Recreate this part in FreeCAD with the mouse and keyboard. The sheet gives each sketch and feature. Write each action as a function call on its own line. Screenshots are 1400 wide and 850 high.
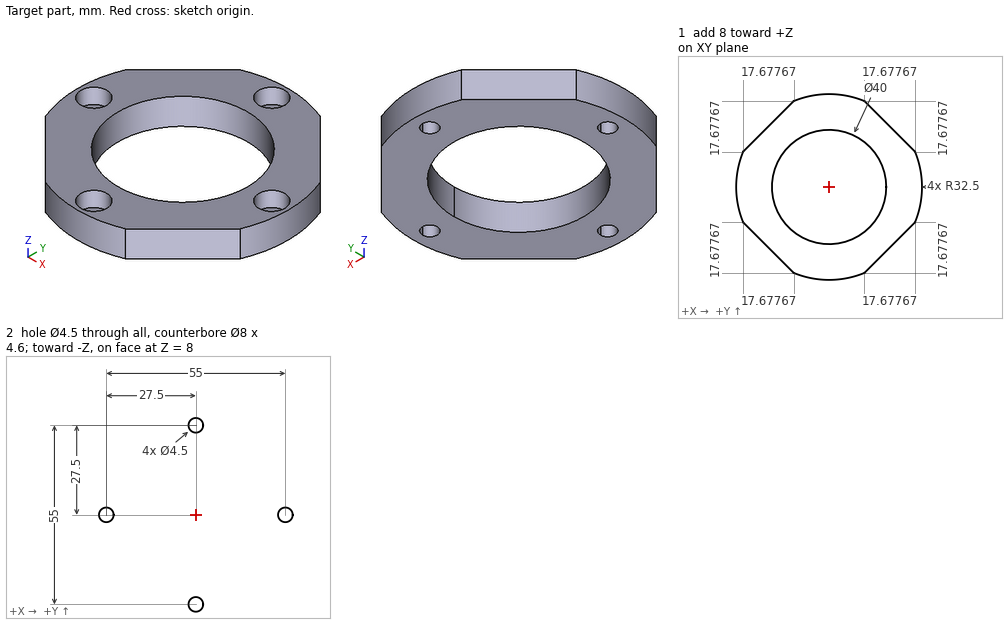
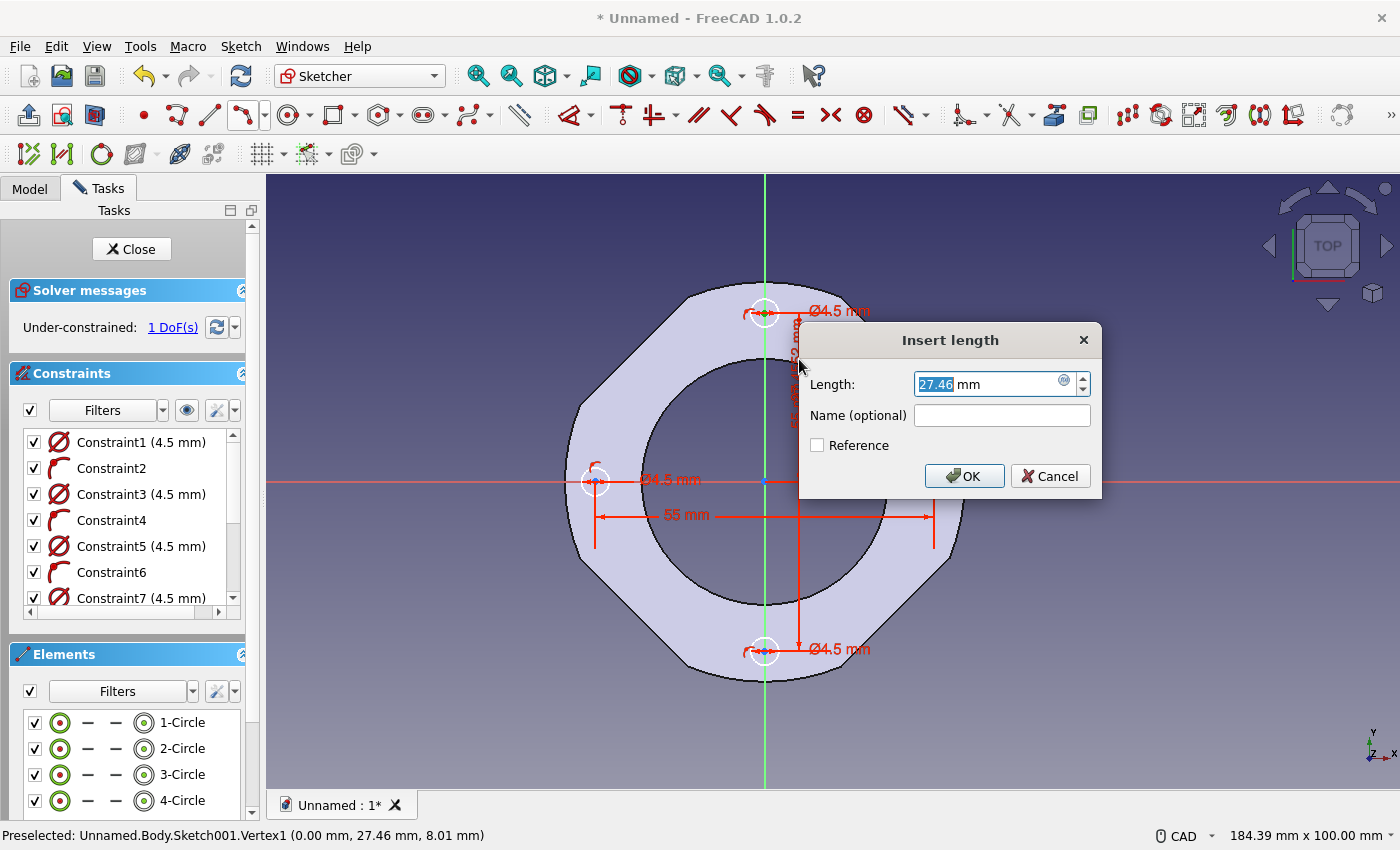
text(27.5)
key(Return)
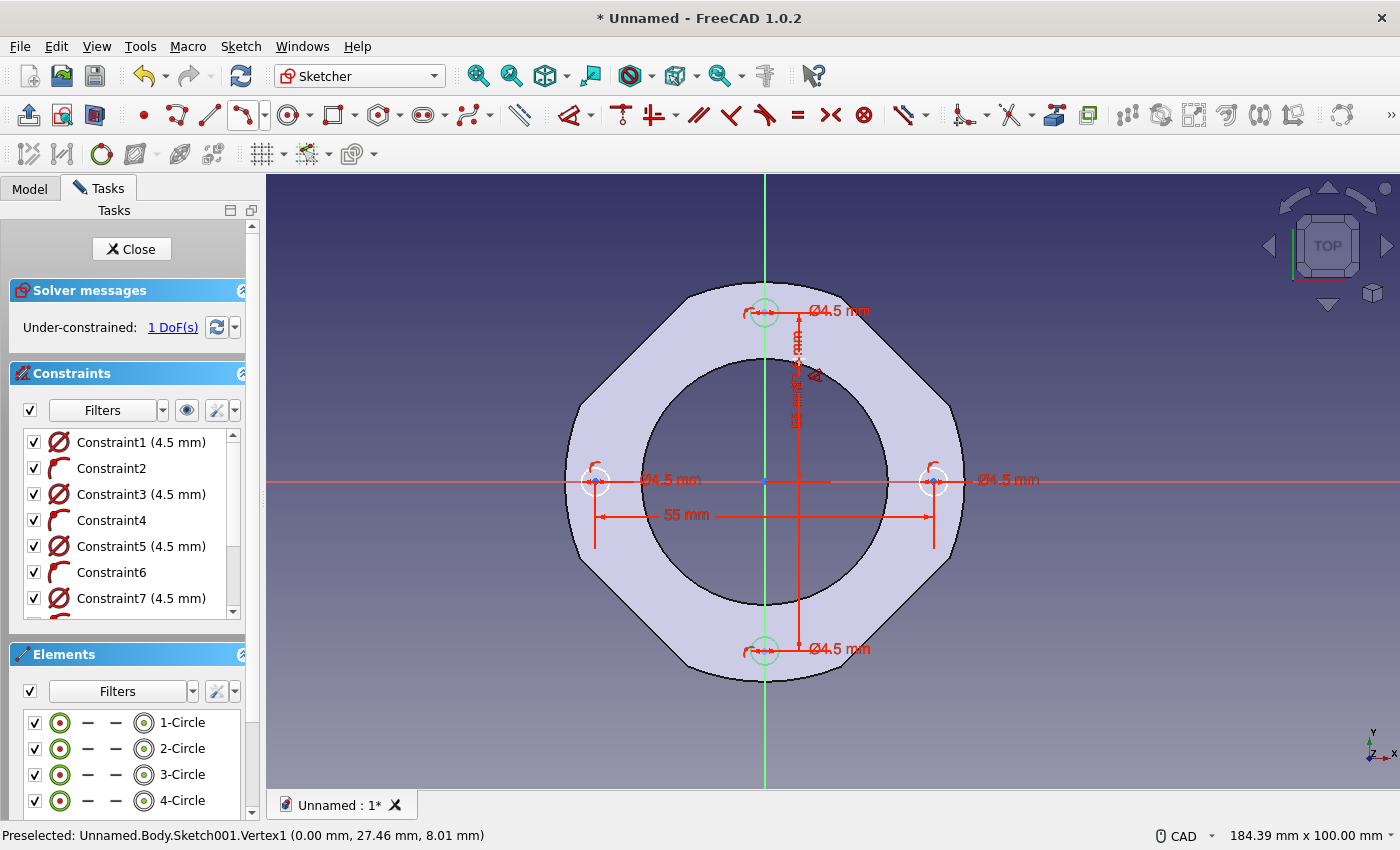
click(595, 482)
click(680, 448)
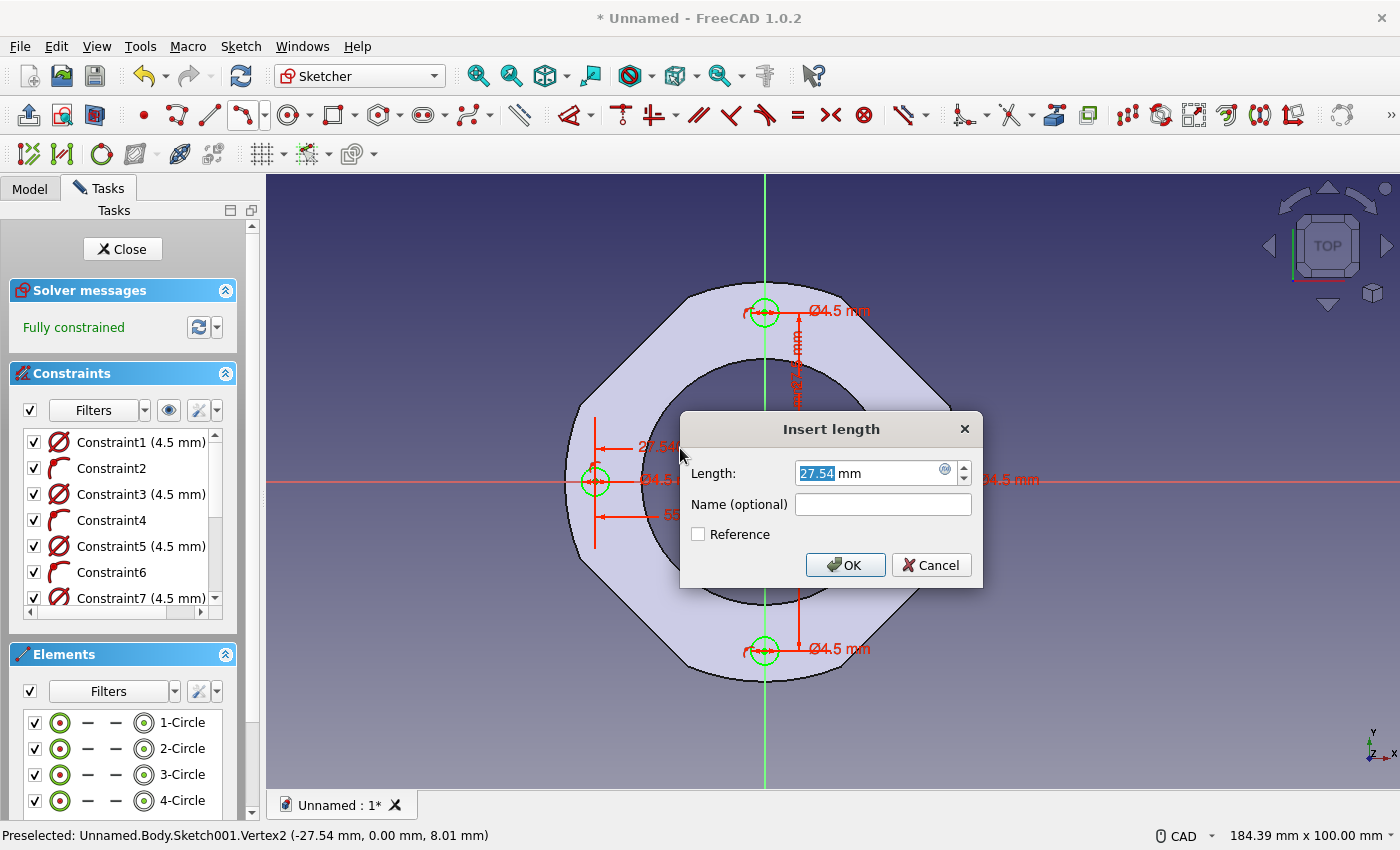
text(27.5)
key(Return)
key(Escape)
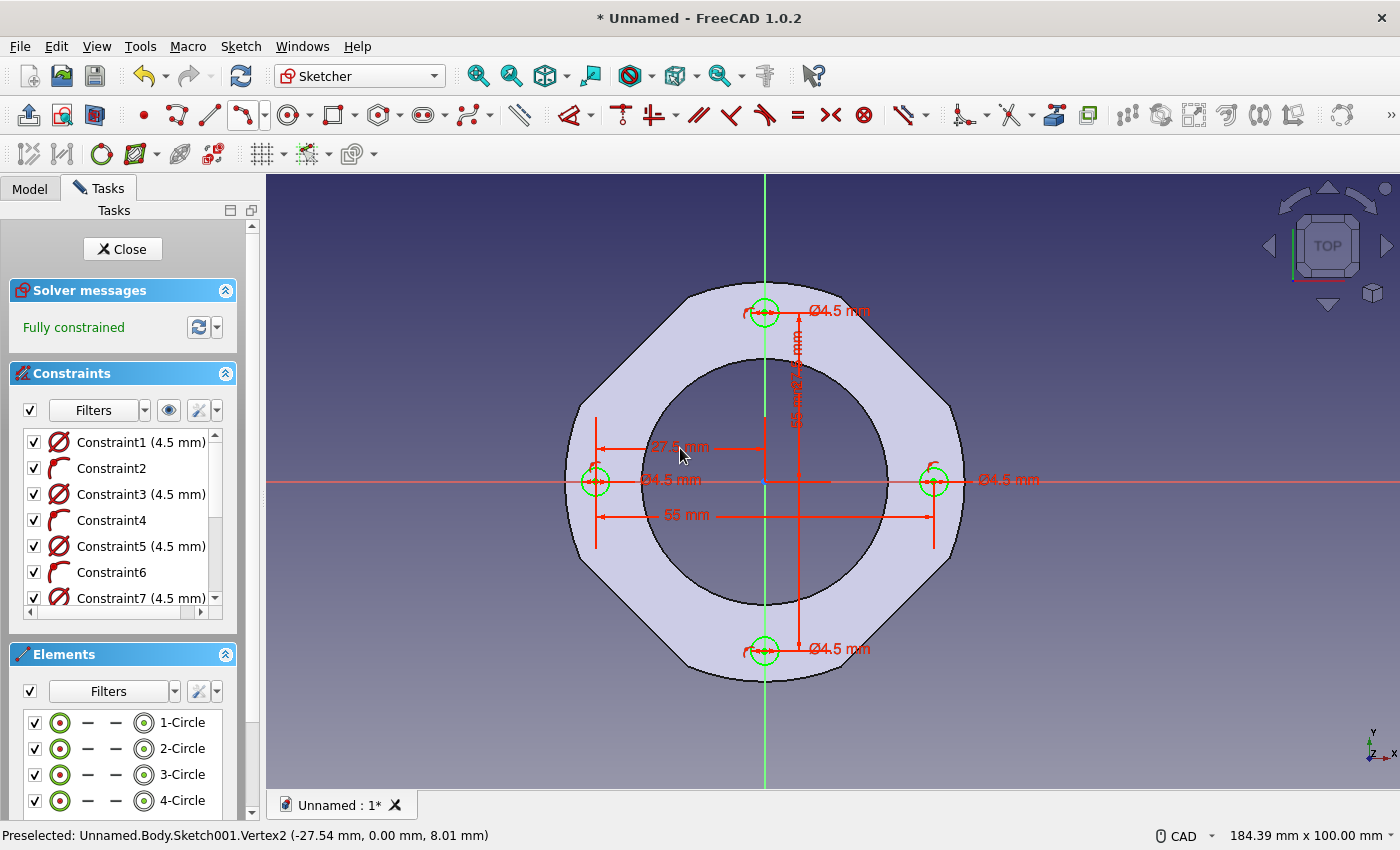
click(123, 249)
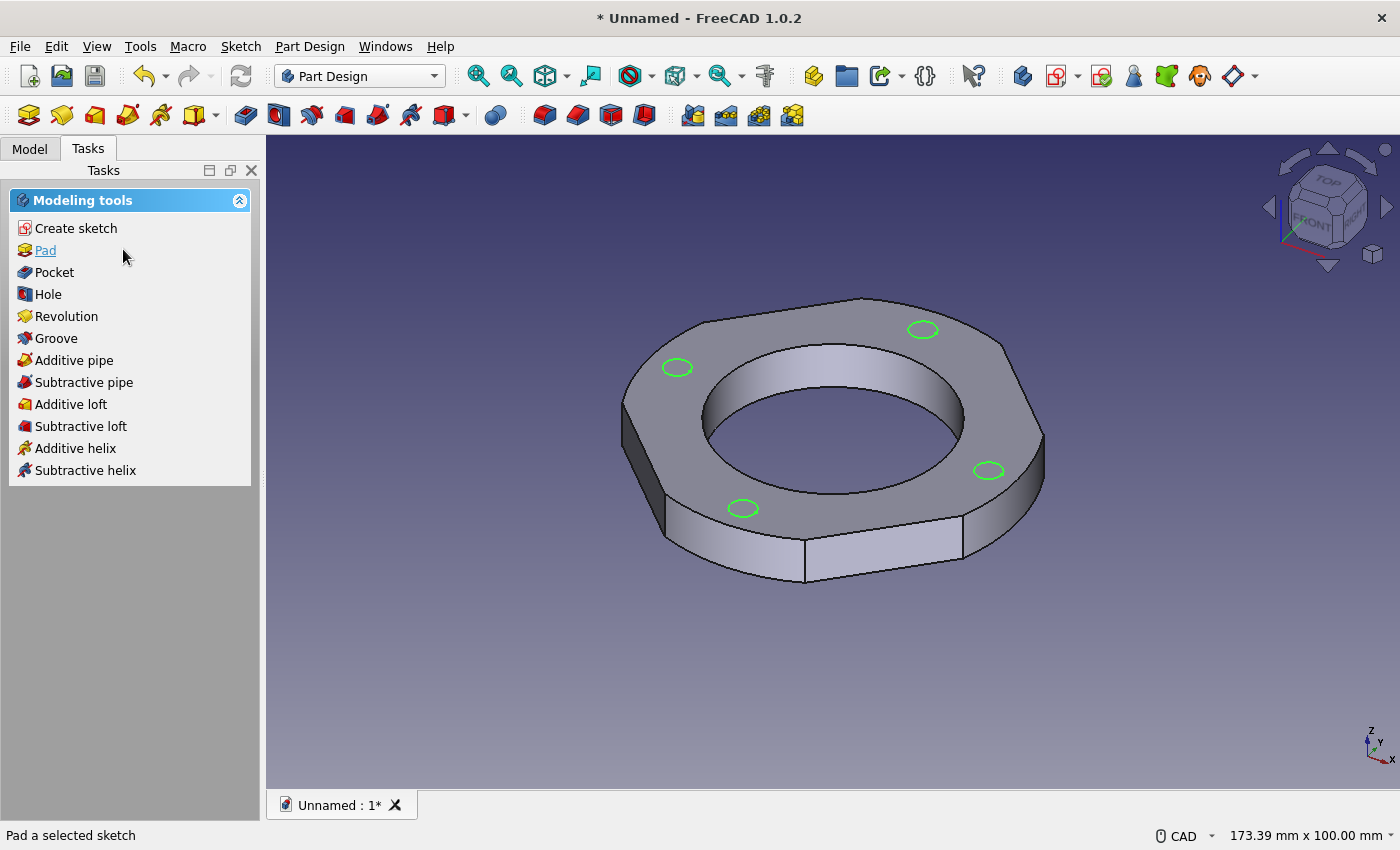
click(279, 116)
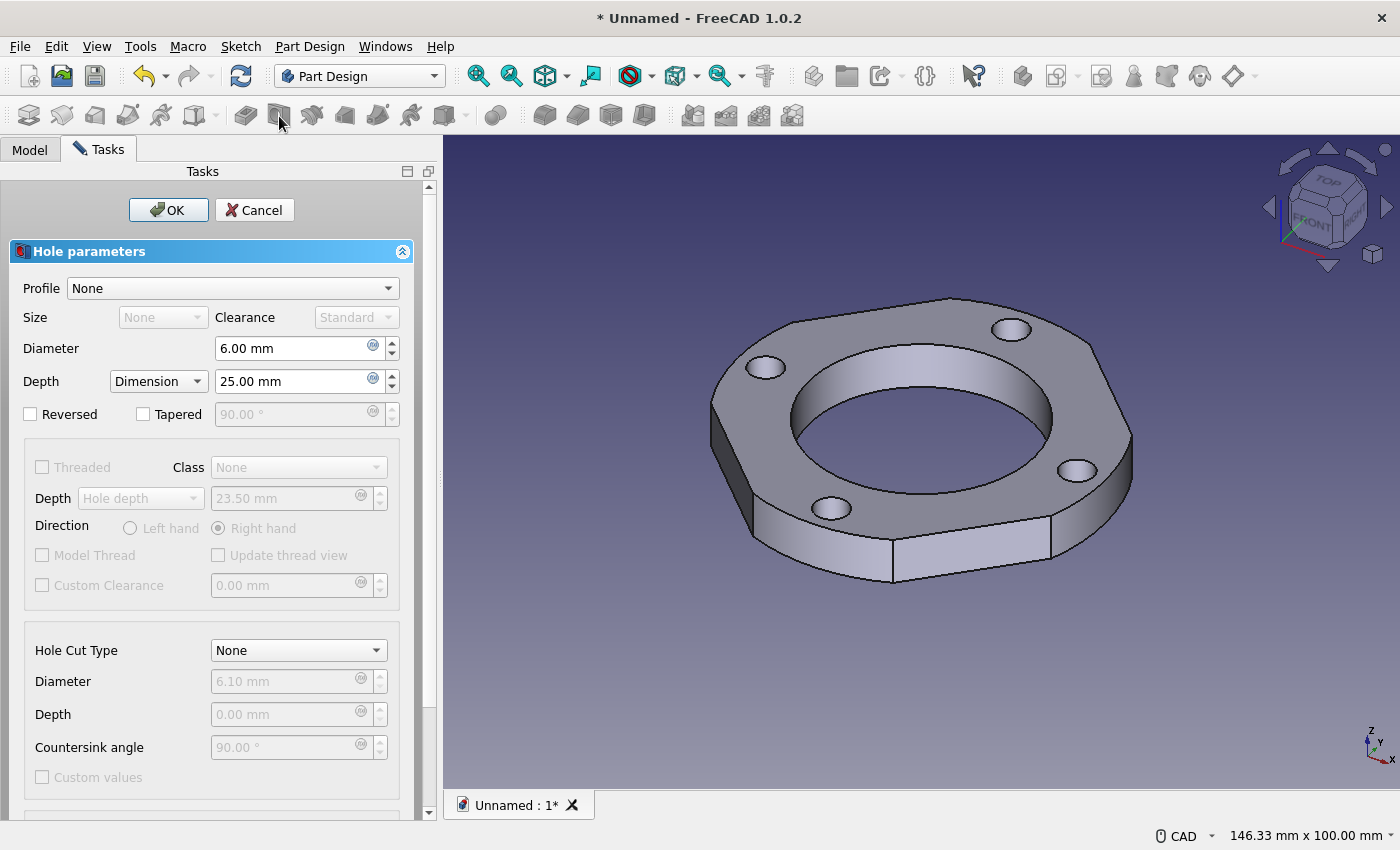
triple_click(300, 348)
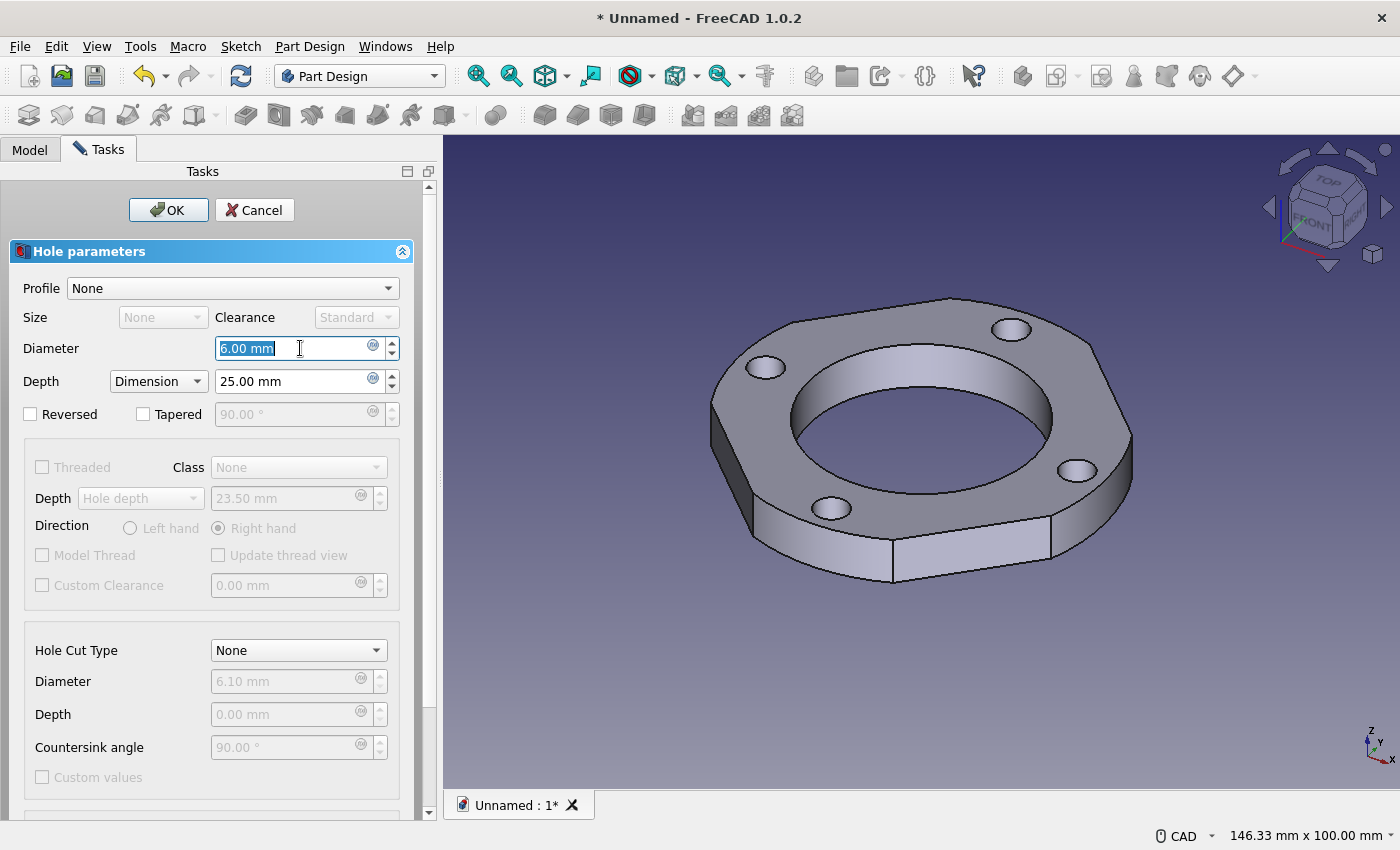
text(4.5)
key(Tab)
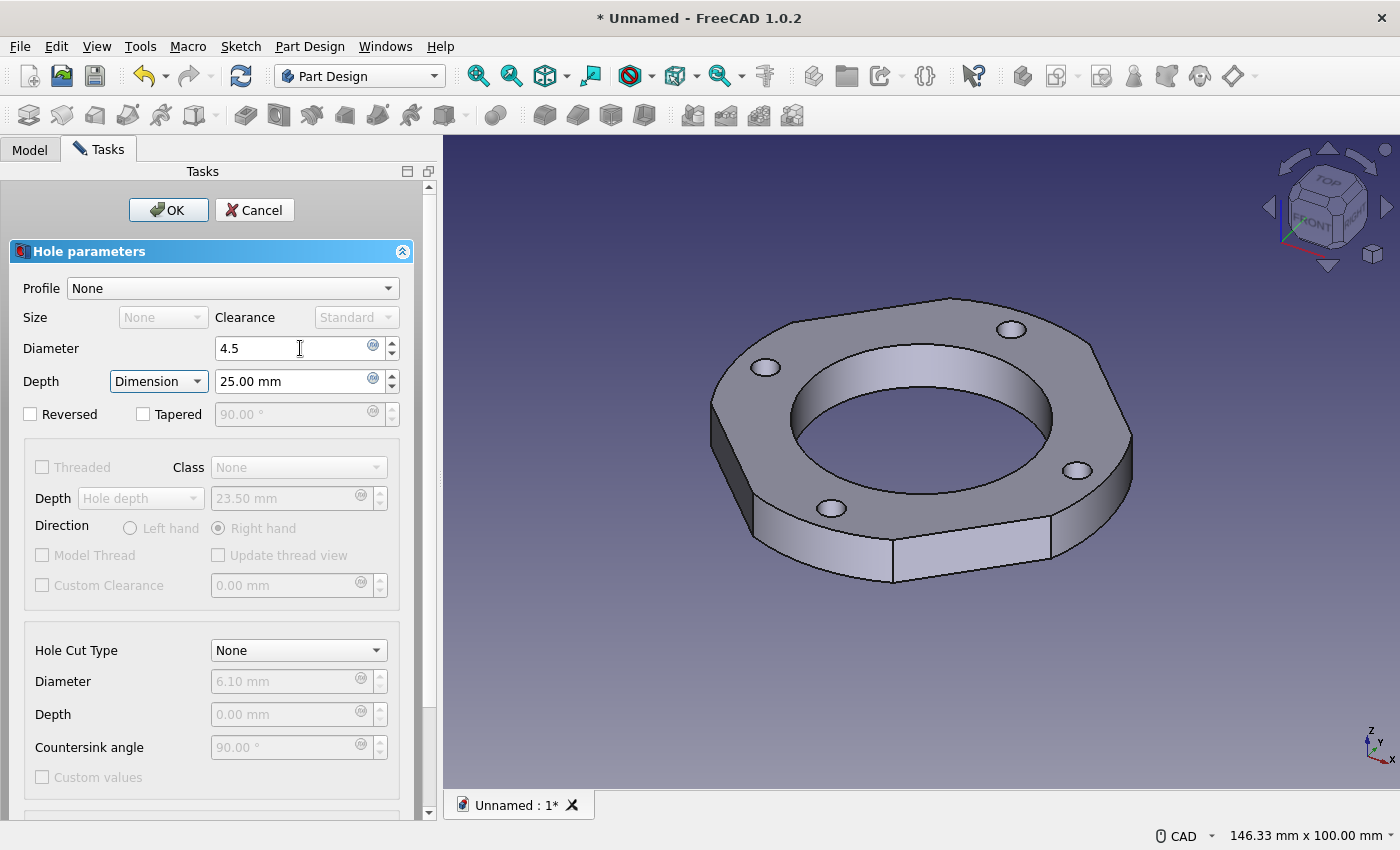
click(160, 382)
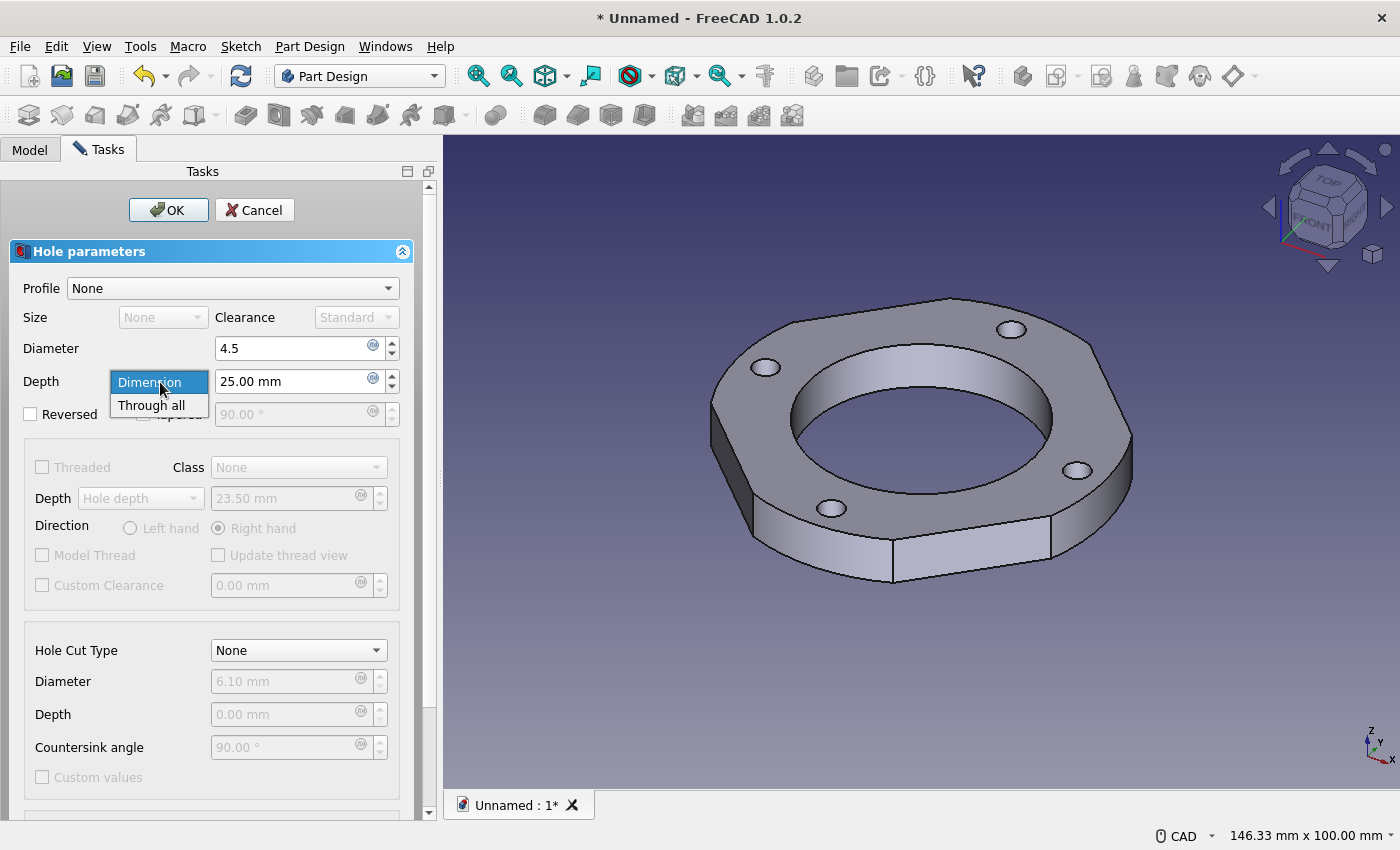
click(158, 406)